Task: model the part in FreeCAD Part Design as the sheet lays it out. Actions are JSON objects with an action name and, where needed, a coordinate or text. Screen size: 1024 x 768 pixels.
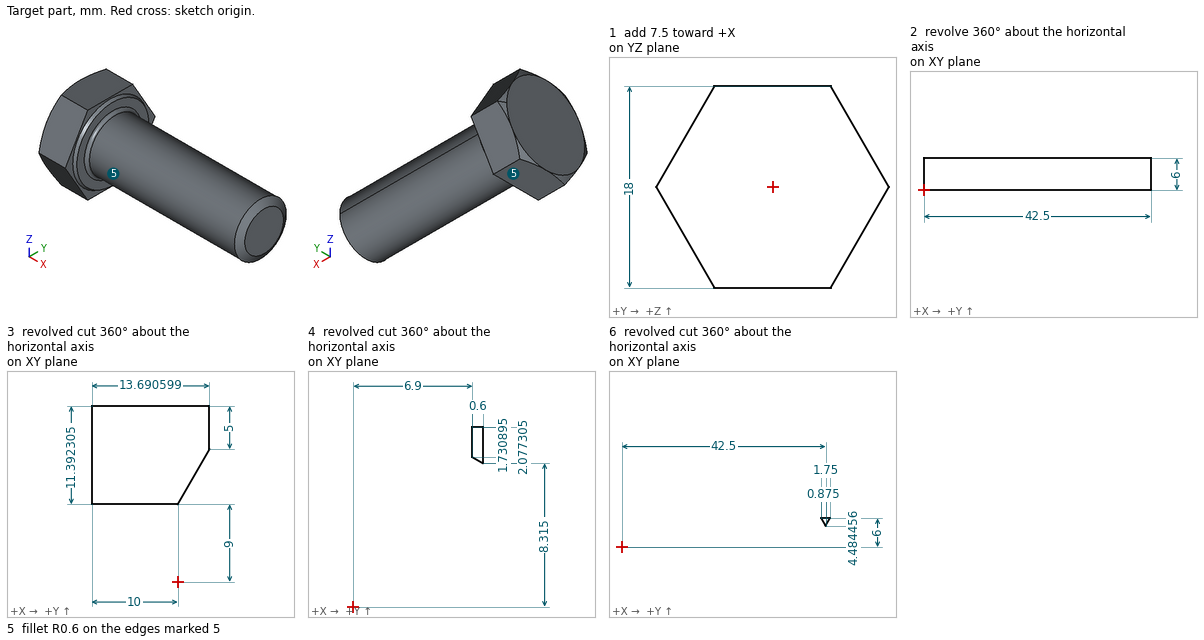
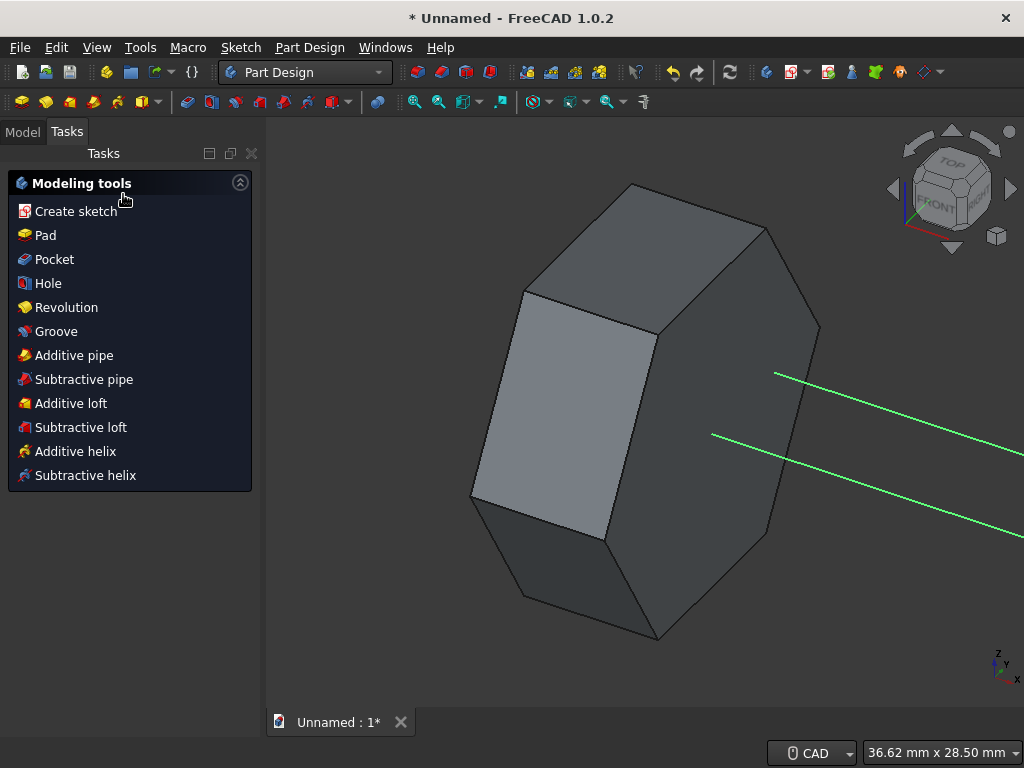
{"action": "left_click", "coordinate": [46, 102]}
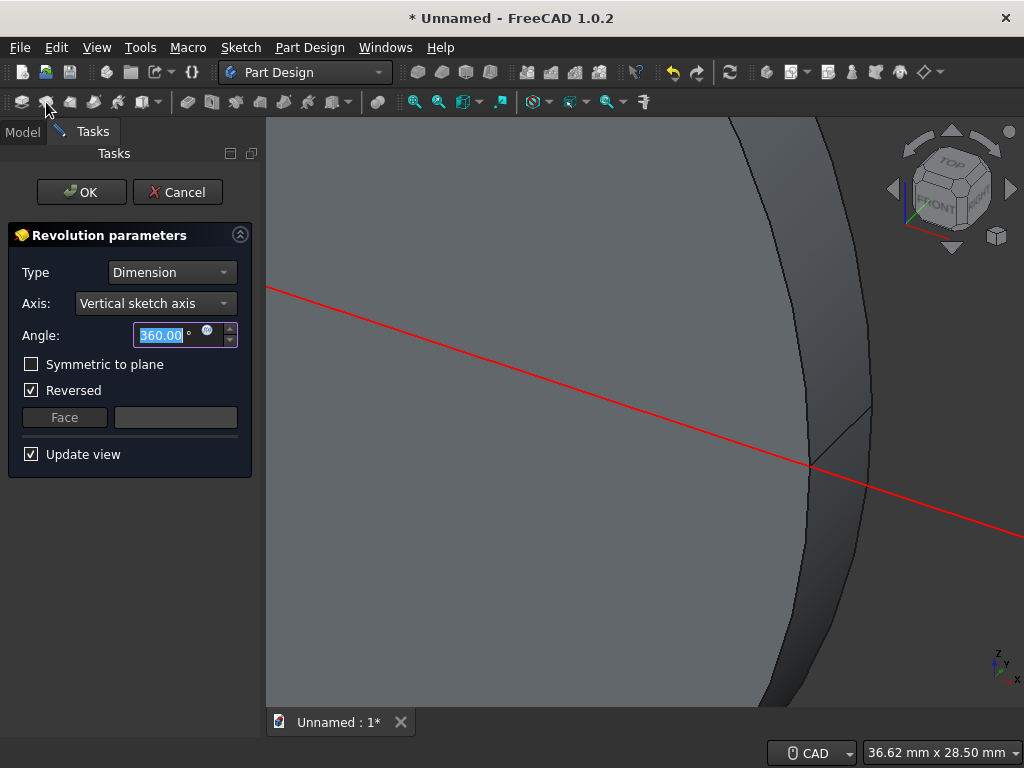
{"action": "left_click", "coordinate": [156, 304]}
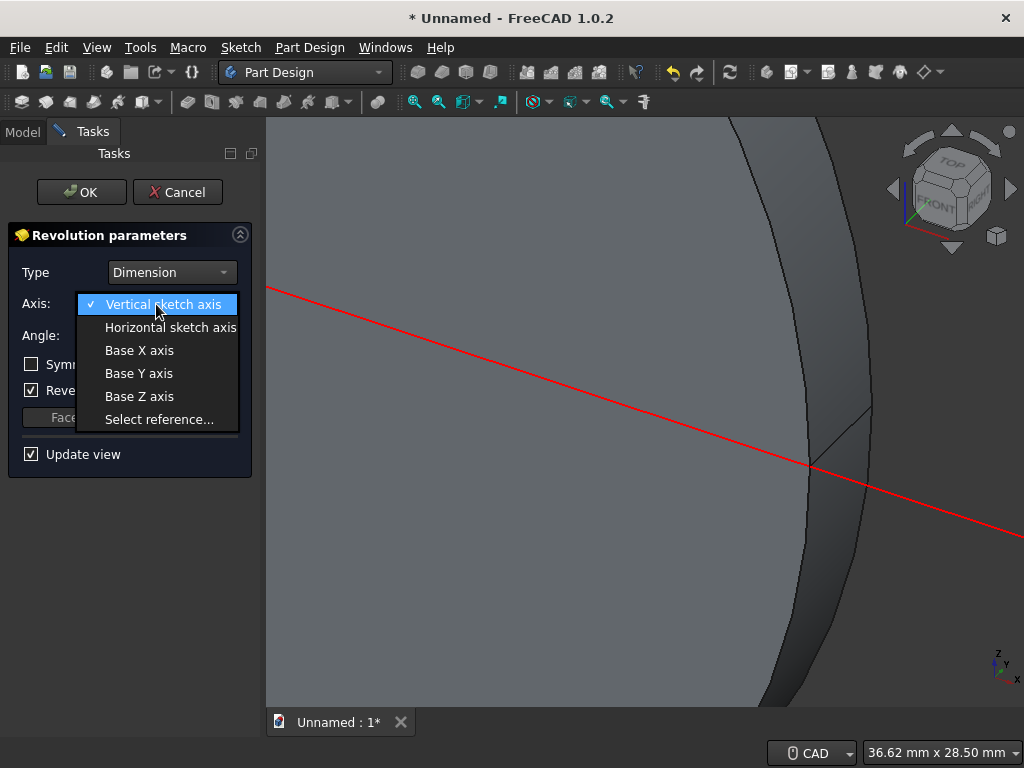
{"action": "left_click", "coordinate": [156, 328]}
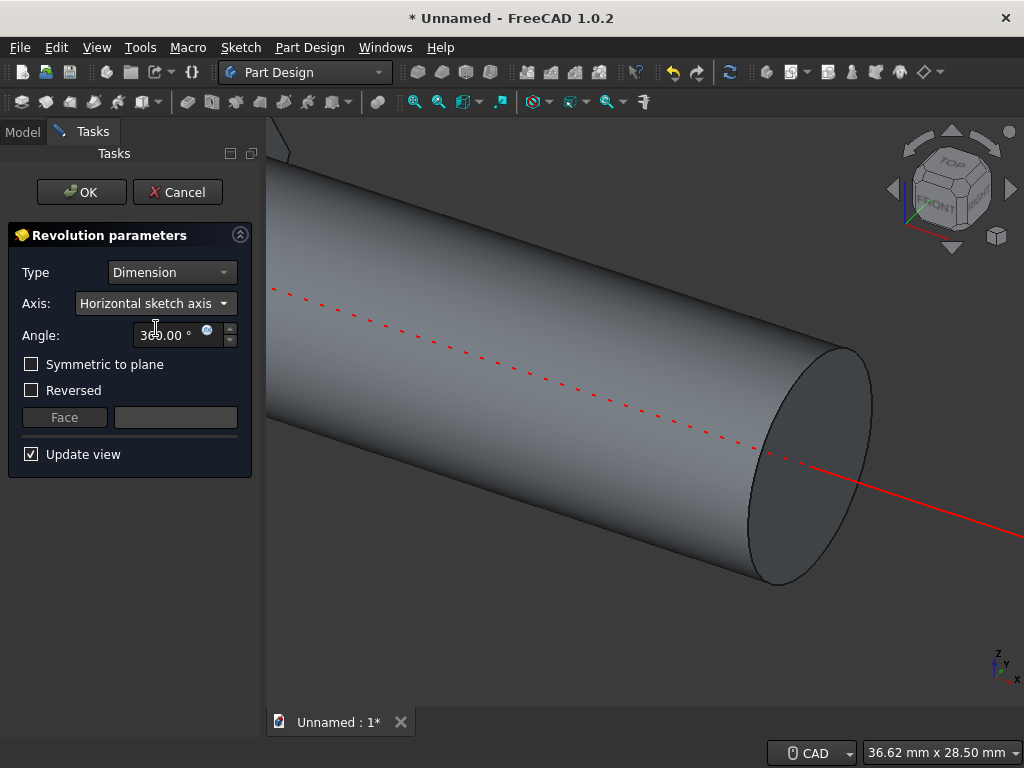
{"action": "left_click", "coordinate": [82, 192]}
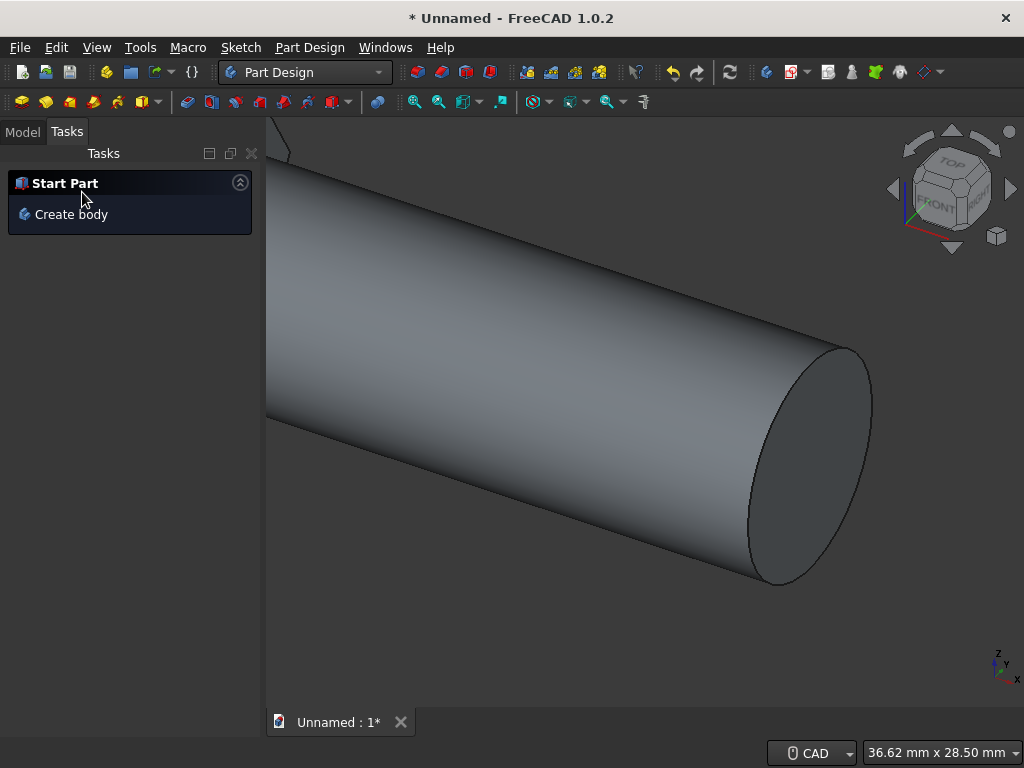
{"action": "left_click", "coordinate": [416, 102]}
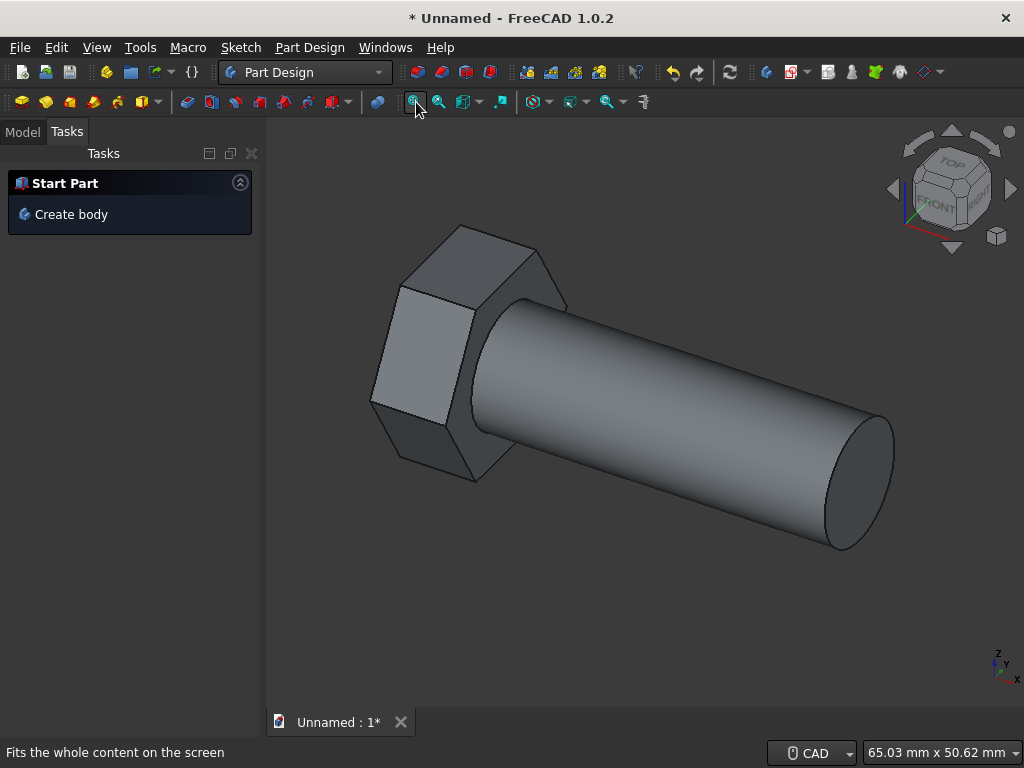
{"action": "left_click", "coordinate": [792, 72]}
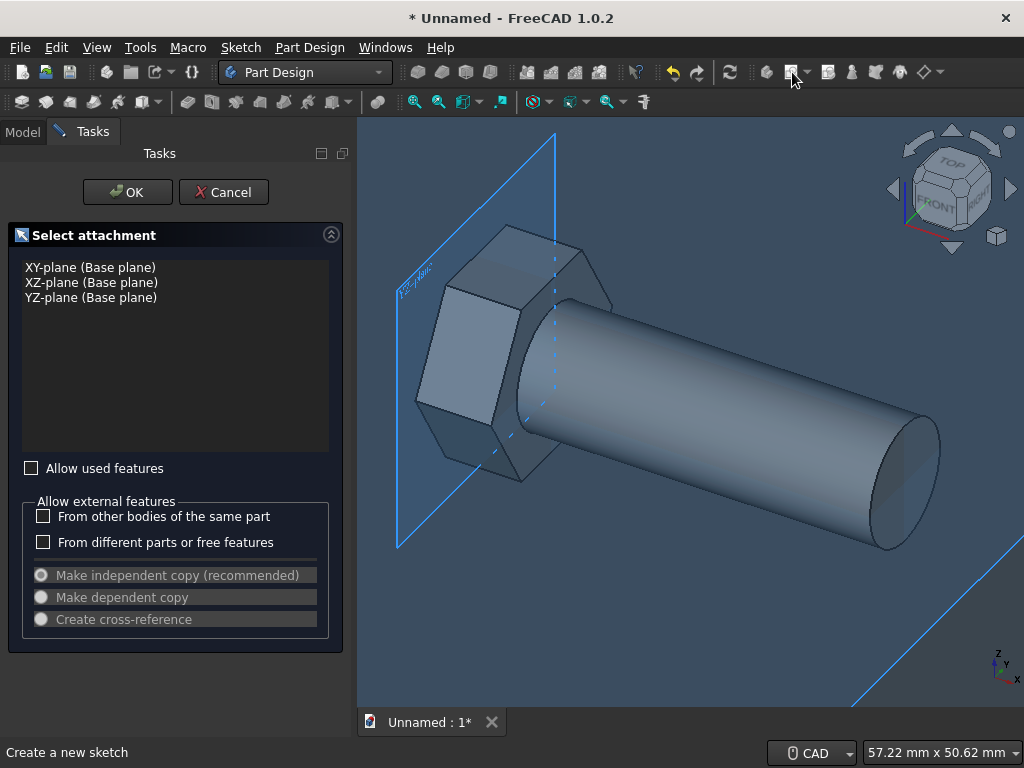
{"action": "left_click", "coordinate": [82, 268]}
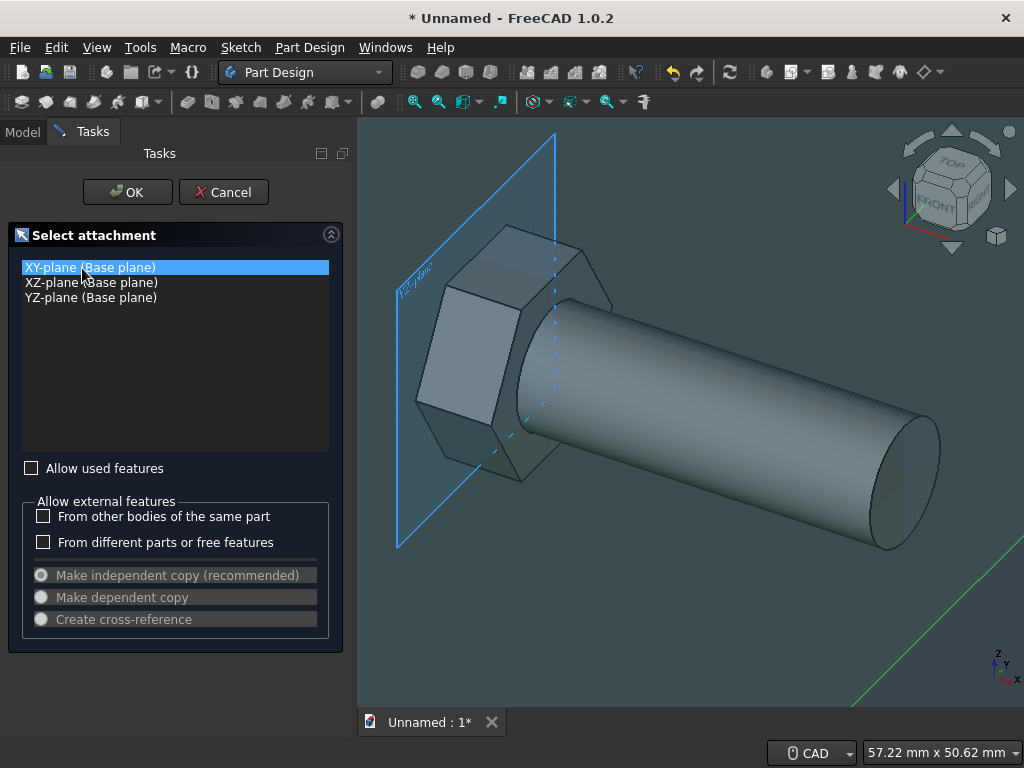
{"action": "left_click", "coordinate": [128, 192]}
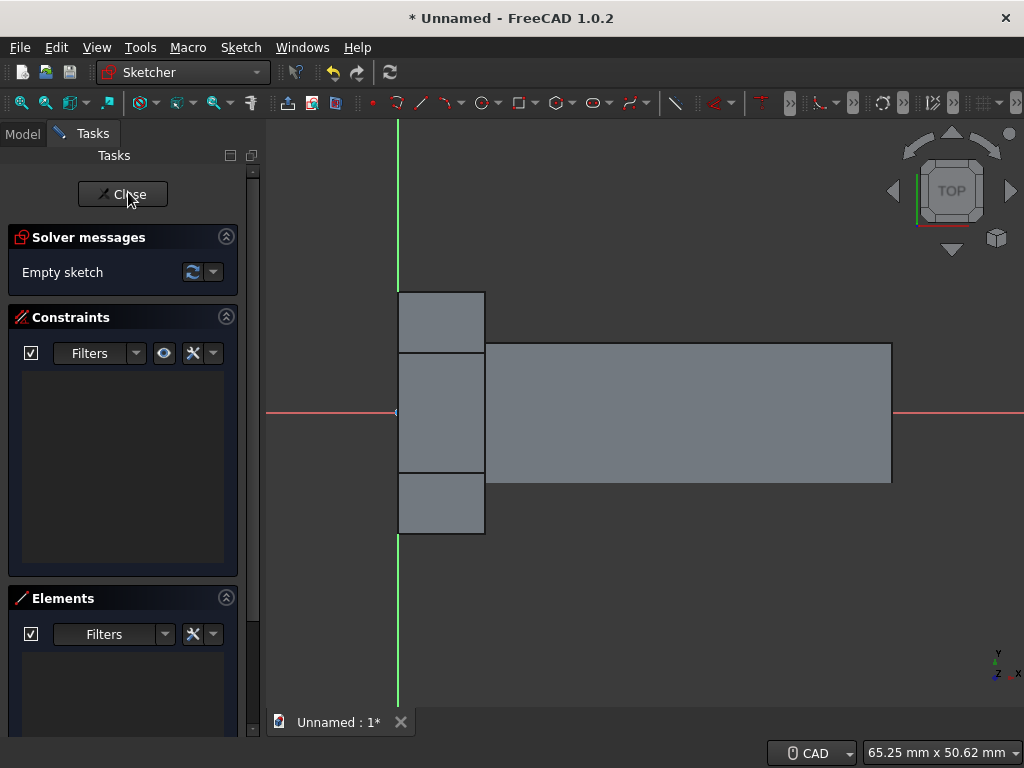
{"action": "left_click", "coordinate": [336, 104]}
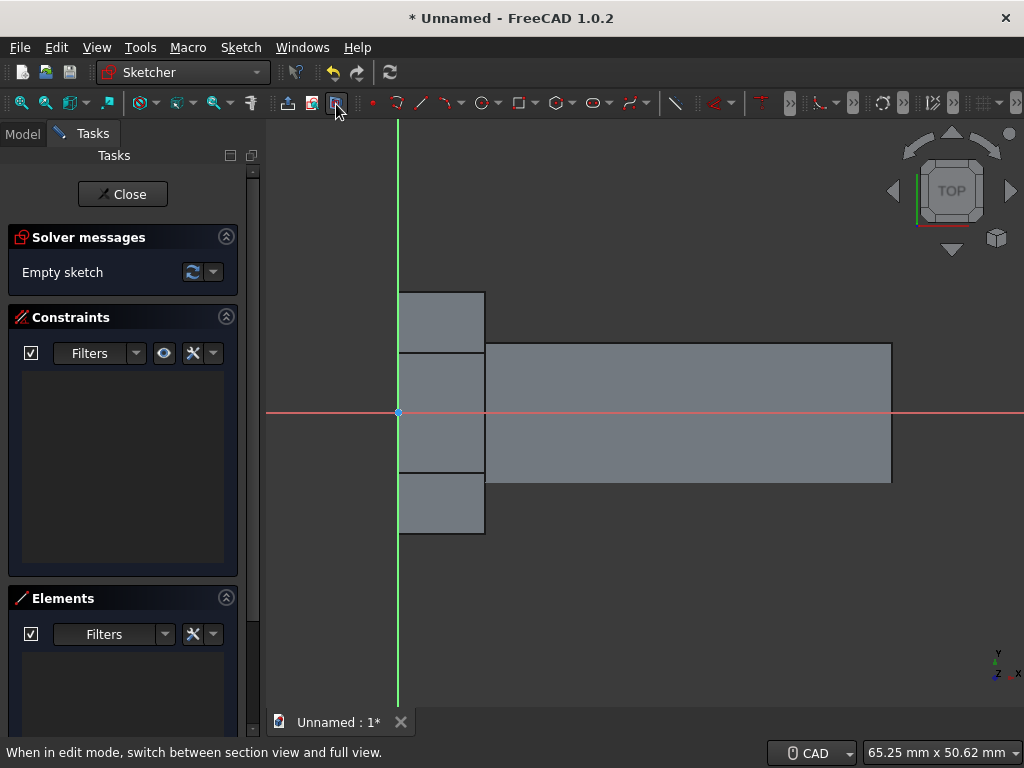
{"action": "scroll", "coordinate": [859, 679], "scroll_direction": "down", "scroll_amount": 1}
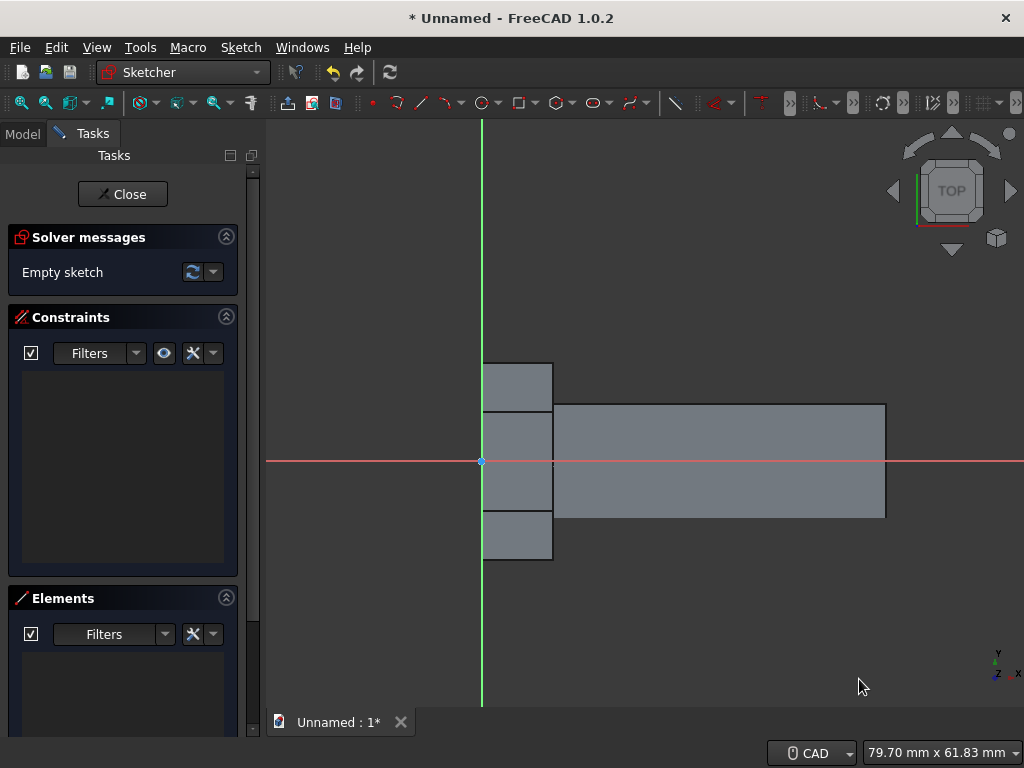
{"action": "scroll", "coordinate": [300, 305], "scroll_direction": "up", "scroll_amount": 3}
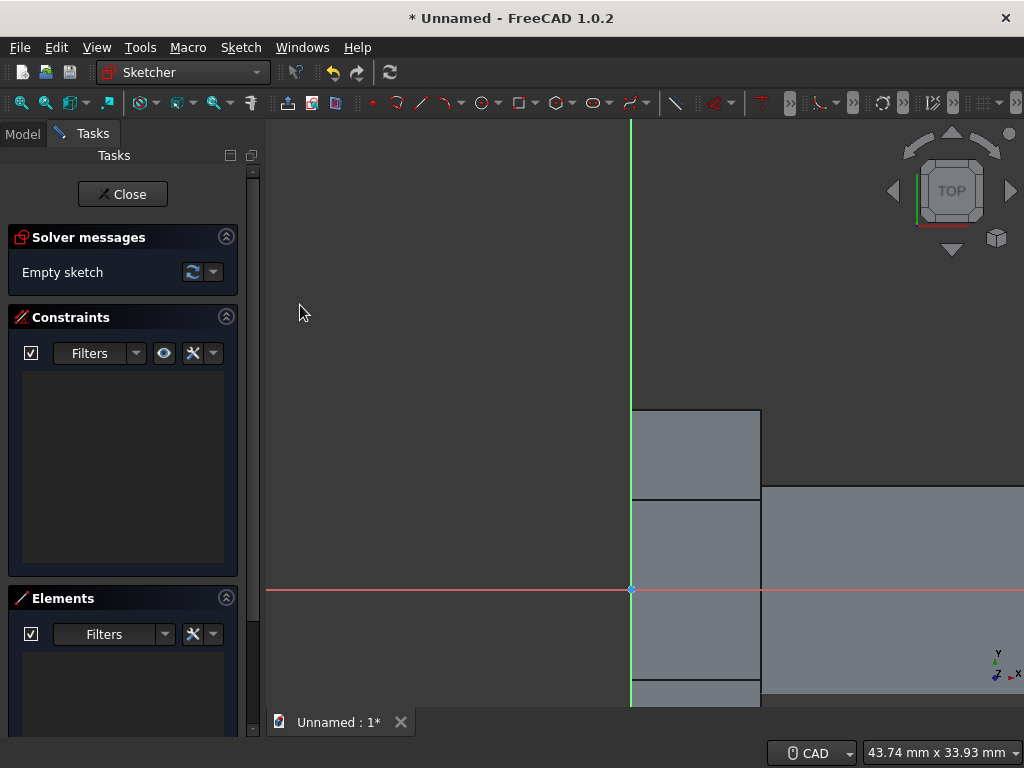
{"action": "left_click", "coordinate": [398, 104]}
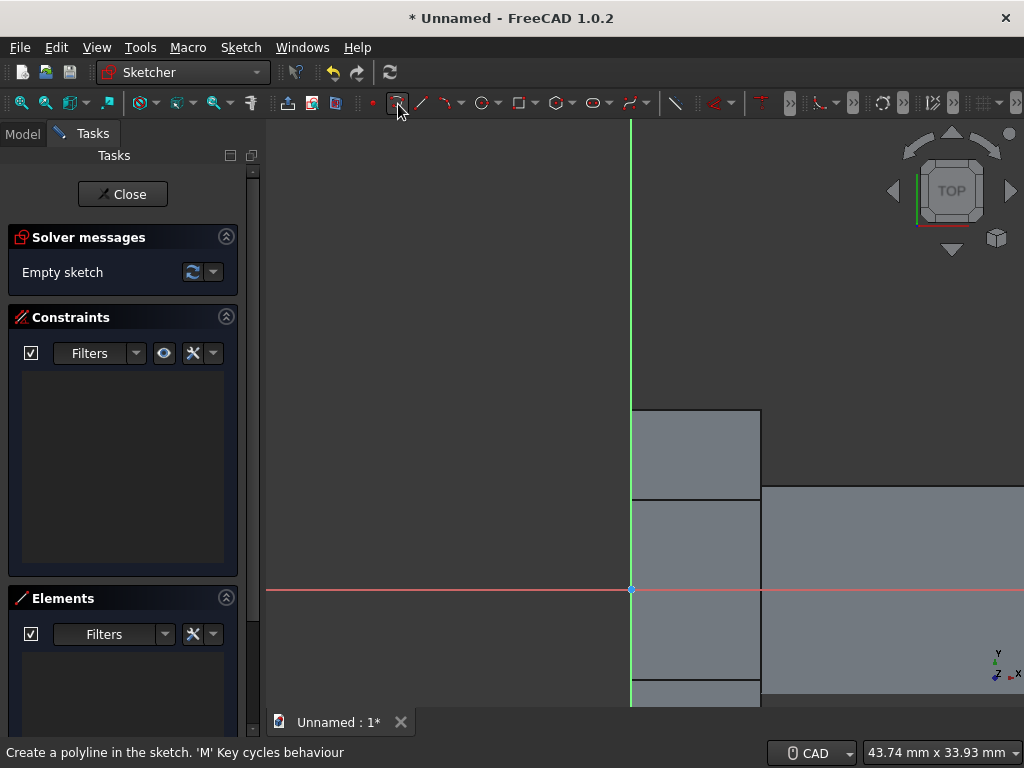
{"action": "left_click", "coordinate": [631, 434]}
{"action": "left_click", "coordinate": [695, 323]}
{"action": "left_click", "coordinate": [695, 236]}
{"action": "left_click", "coordinate": [458, 236]}
{"action": "left_click", "coordinate": [458, 434]}
{"action": "left_click", "coordinate": [631, 435]}
{"action": "key", "text": "Escape"}
{"action": "key", "text": "Escape"}